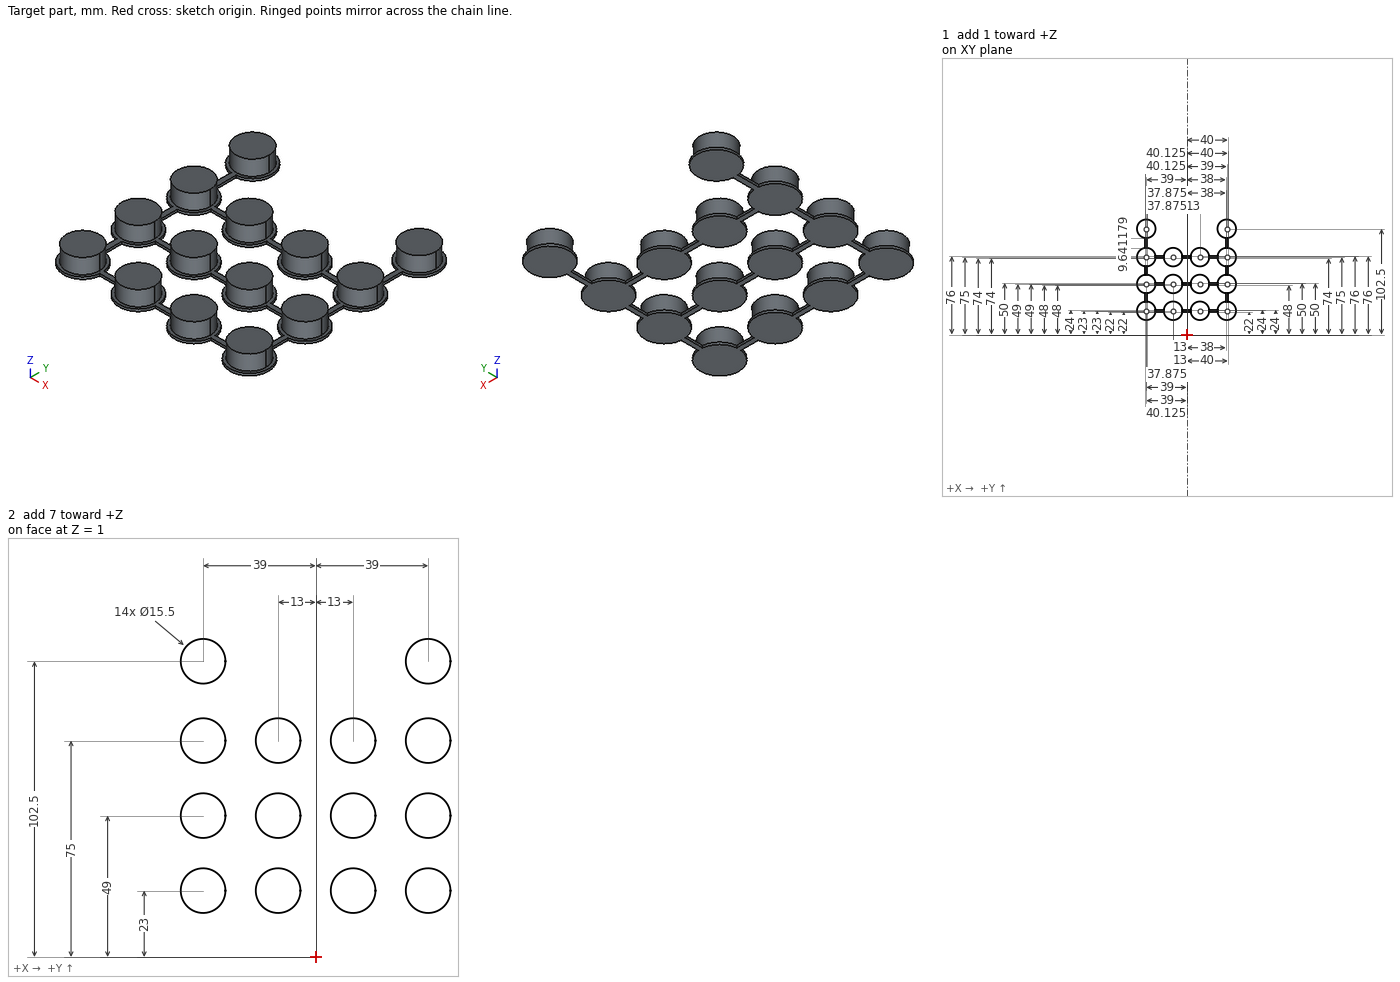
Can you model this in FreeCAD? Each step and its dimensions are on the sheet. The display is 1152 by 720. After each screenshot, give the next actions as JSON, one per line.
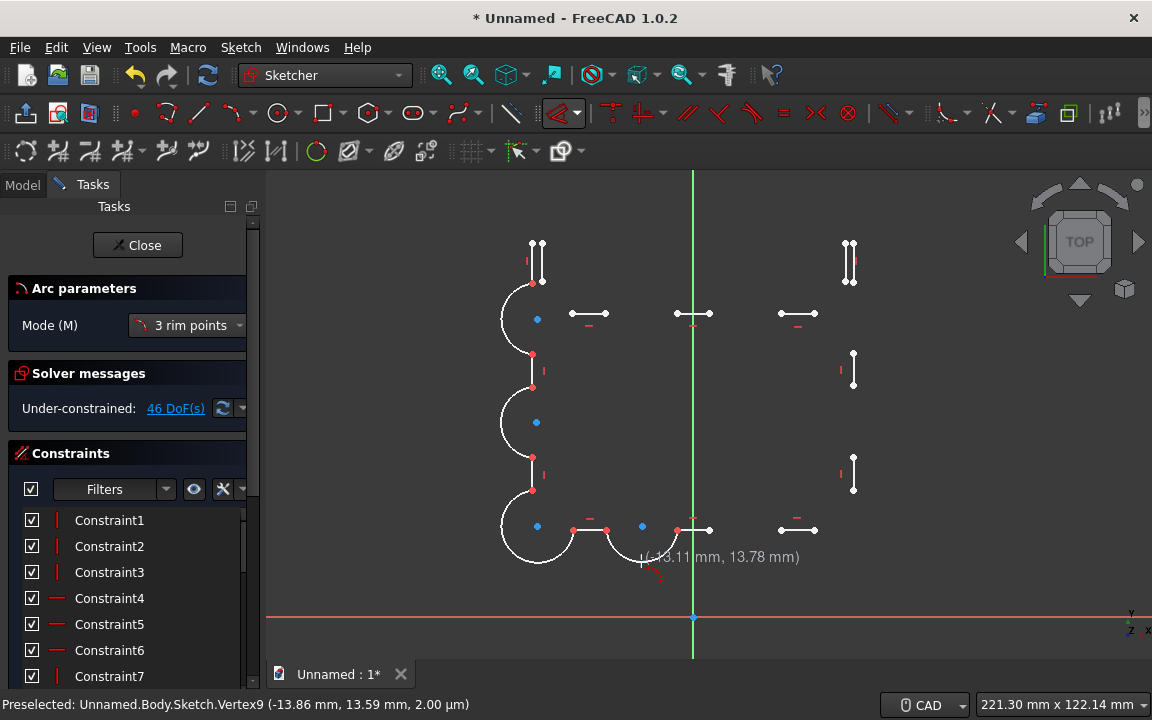
{"action": "left_click", "coordinate": [710, 530]}
{"action": "left_click", "coordinate": [781, 530]}
{"action": "left_click", "coordinate": [746, 561]}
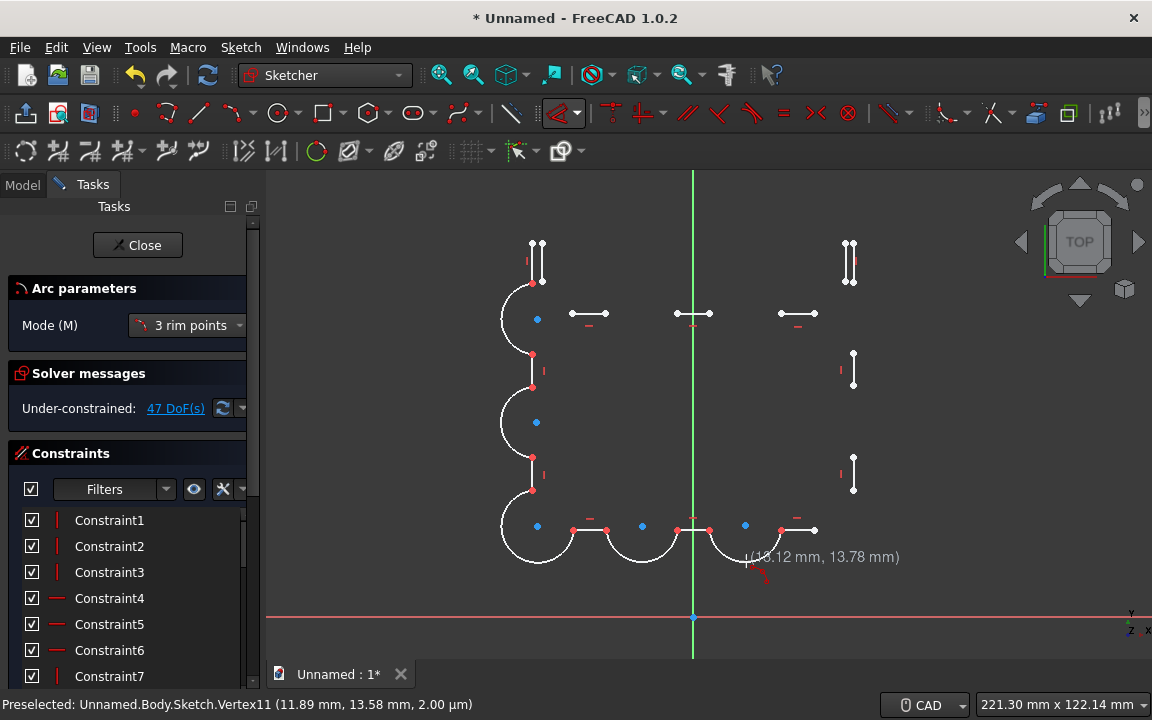
{"action": "left_click", "coordinate": [814, 530]}
{"action": "left_click", "coordinate": [854, 490]}
{"action": "left_click", "coordinate": [875, 551]}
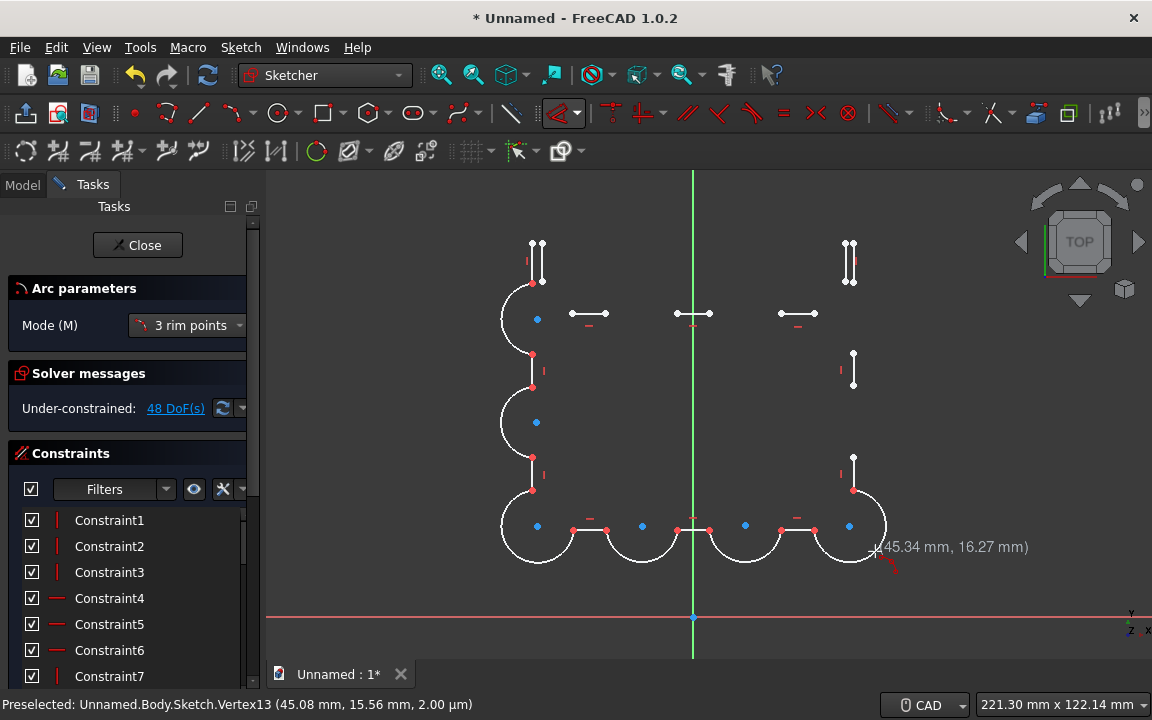
{"action": "left_click", "coordinate": [854, 457]}
{"action": "left_click", "coordinate": [854, 386]}
{"action": "left_click", "coordinate": [886, 421]}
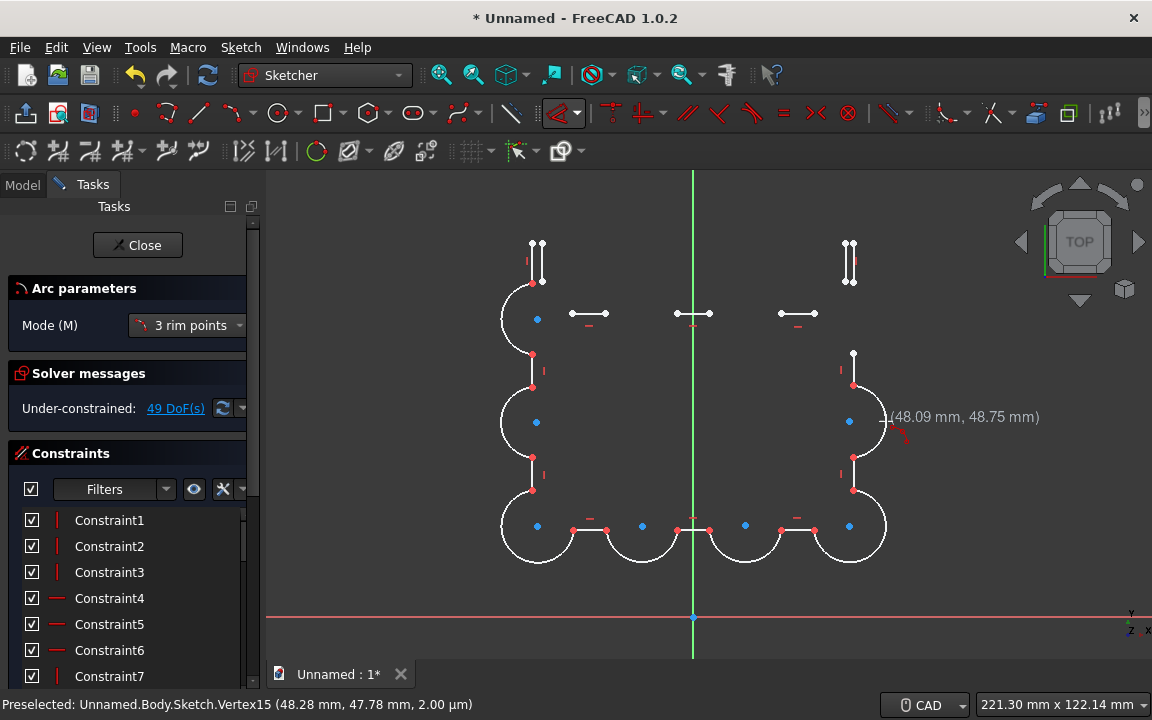
{"action": "left_click", "coordinate": [854, 354]}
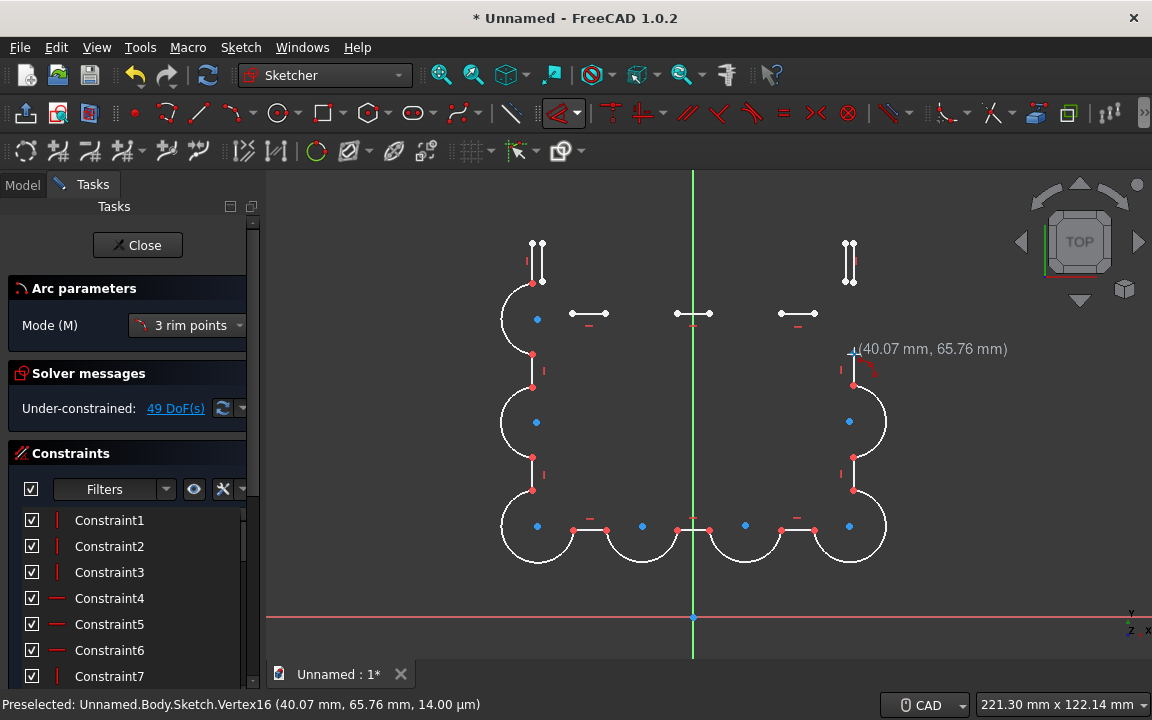
{"action": "scroll", "coordinate": [854, 281], "scroll_direction": "up", "scroll_amount": 4}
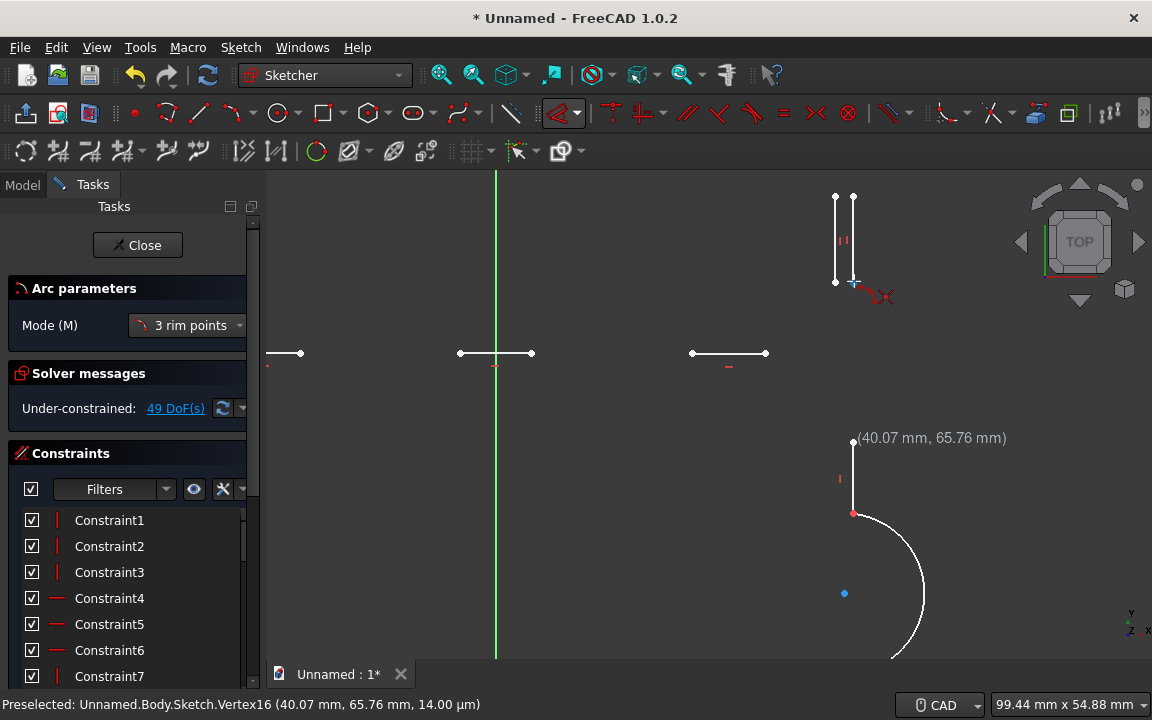
{"action": "left_click", "coordinate": [853, 283]}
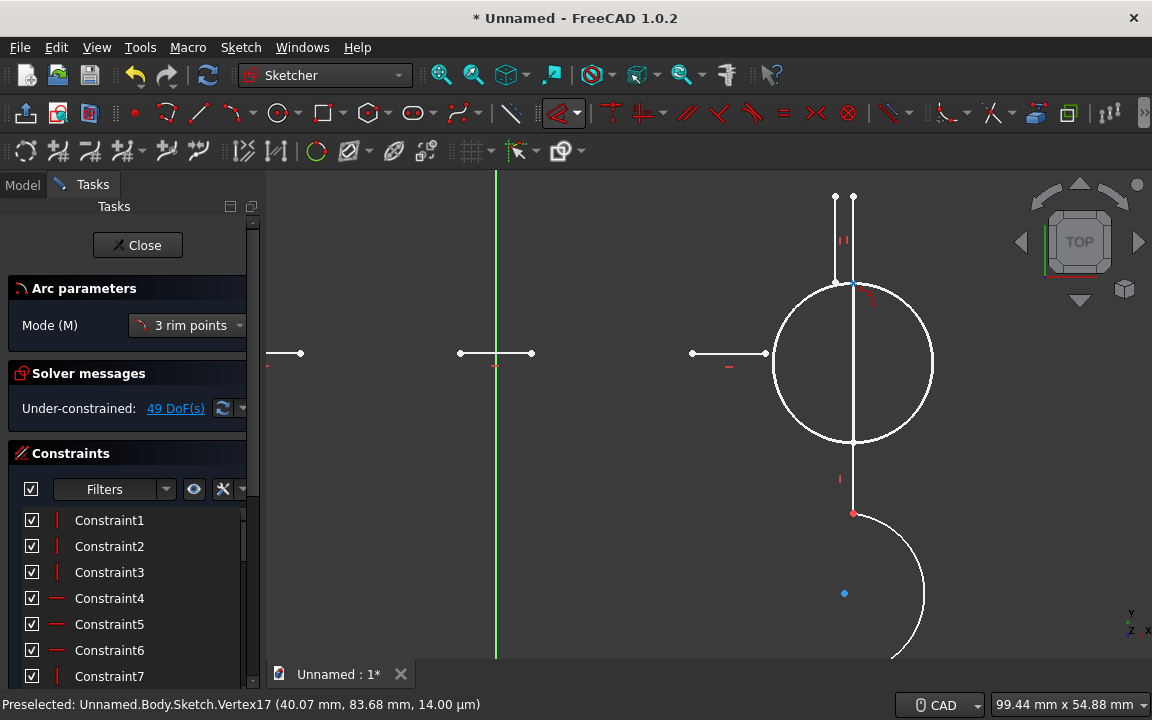
{"action": "scroll", "coordinate": [703, 364], "scroll_direction": "down", "scroll_amount": 6}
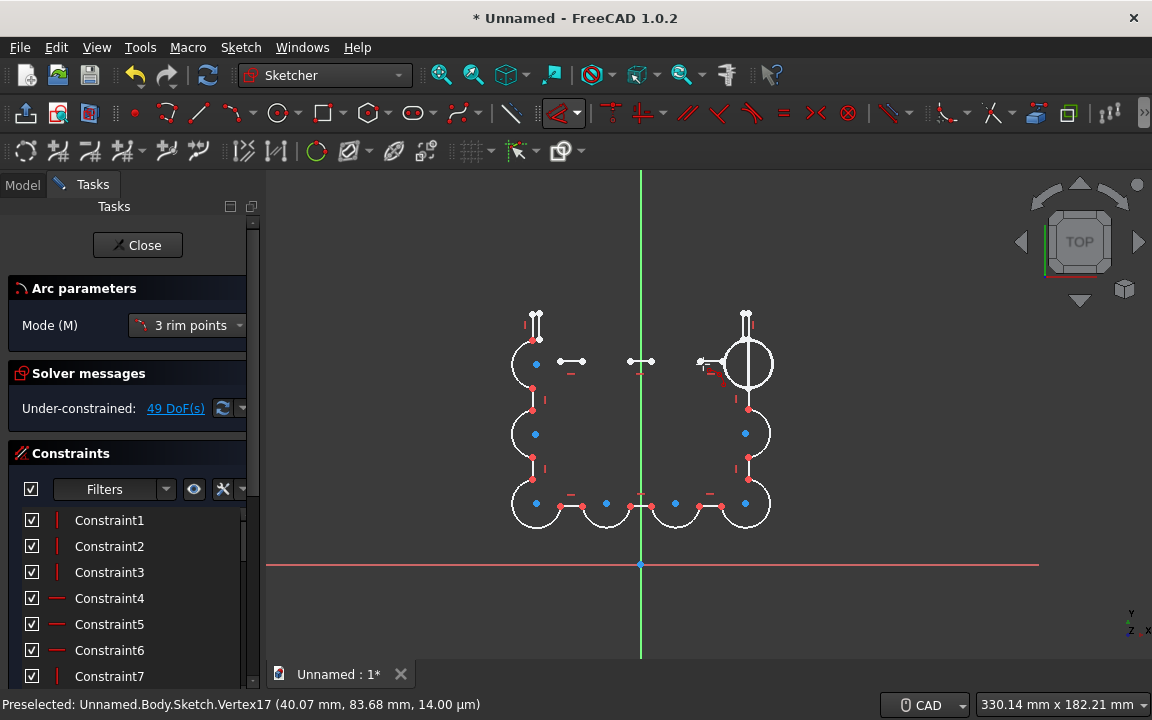
{"action": "left_click", "coordinate": [770, 363]}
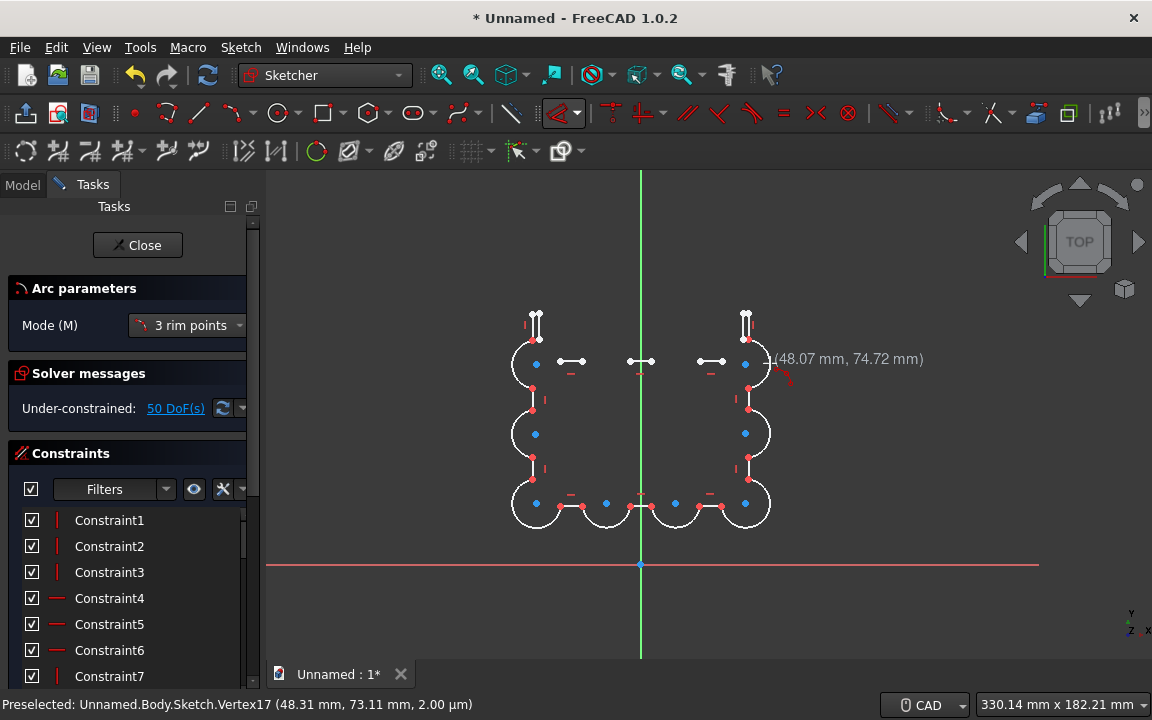
{"action": "scroll", "coordinate": [748, 313], "scroll_direction": "up", "scroll_amount": 6}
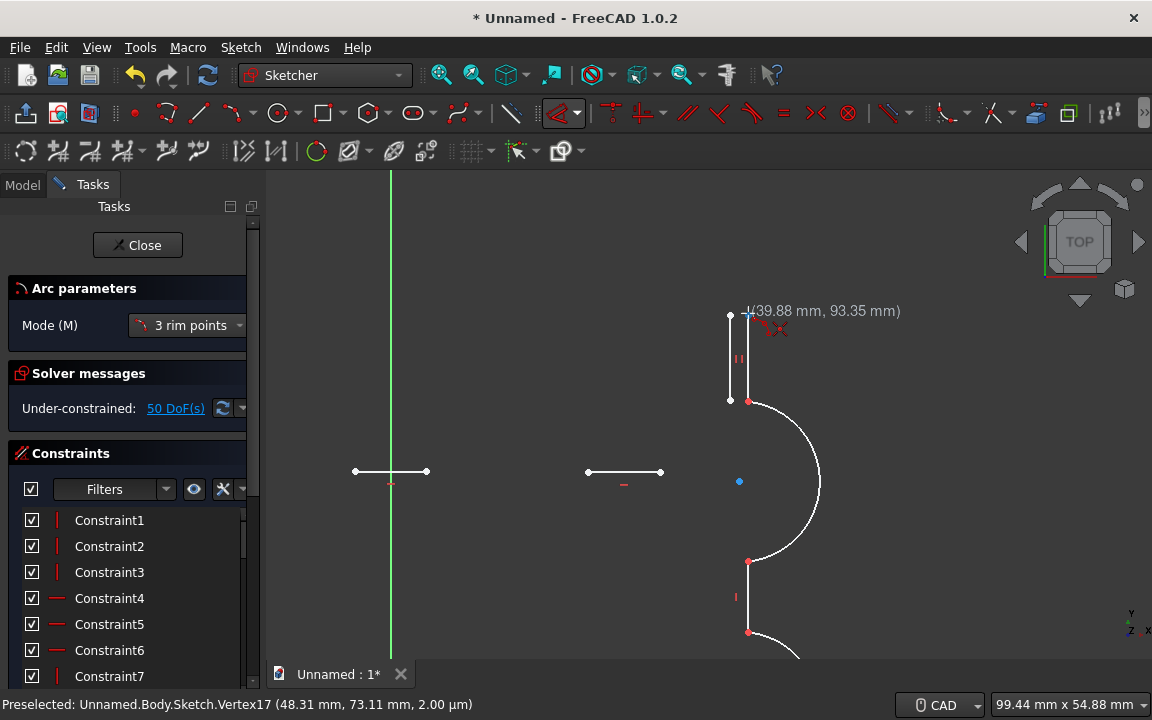
{"action": "left_click", "coordinate": [748, 315]}
{"action": "left_click", "coordinate": [730, 315]}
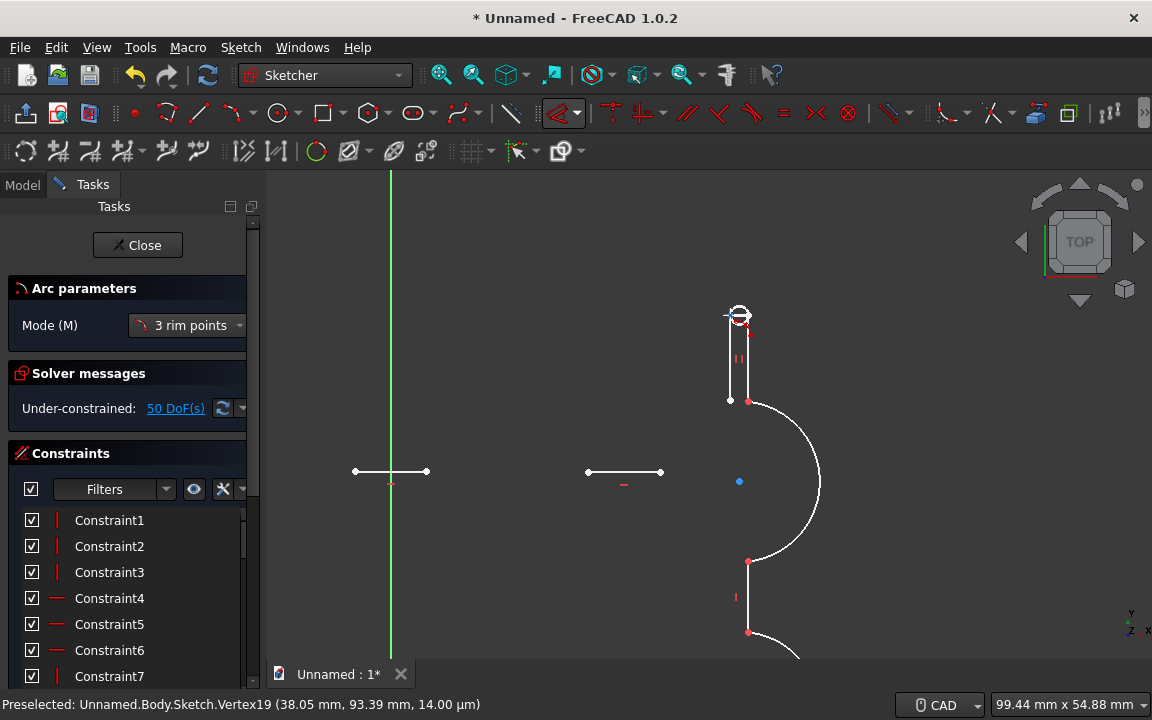
{"action": "scroll", "coordinate": [748, 313], "scroll_direction": "down", "scroll_amount": 6}